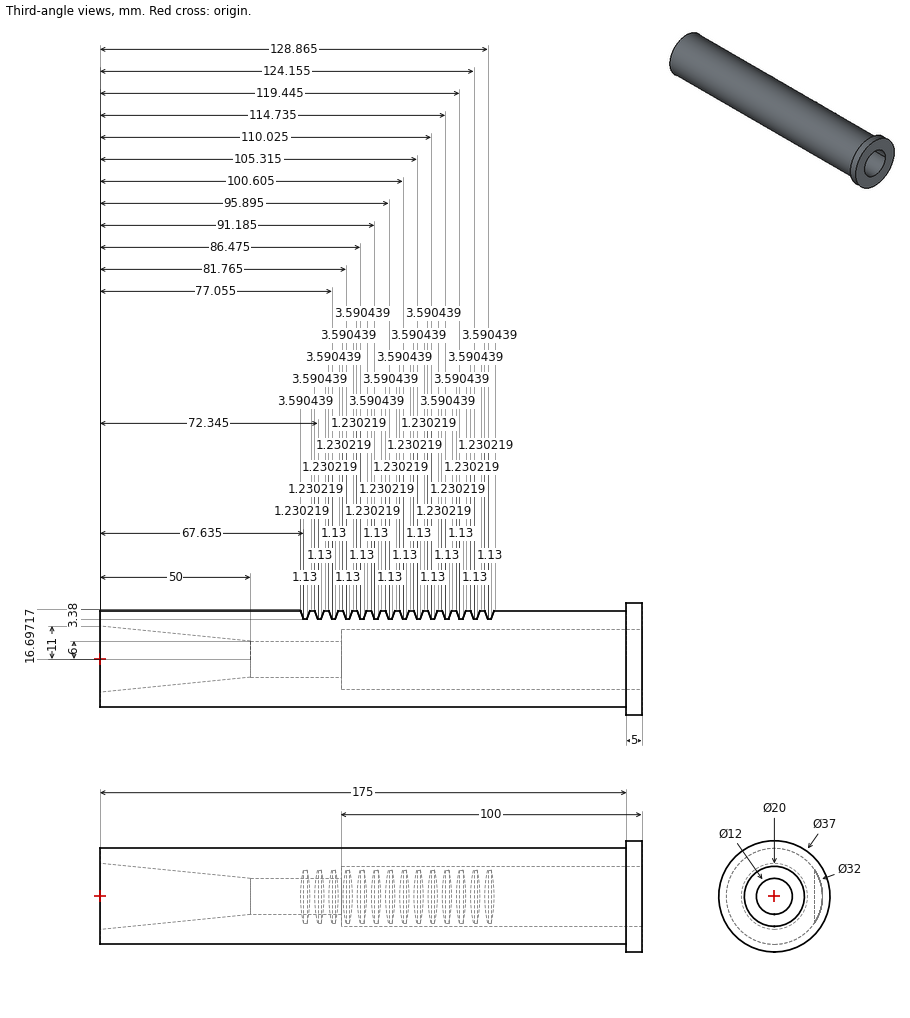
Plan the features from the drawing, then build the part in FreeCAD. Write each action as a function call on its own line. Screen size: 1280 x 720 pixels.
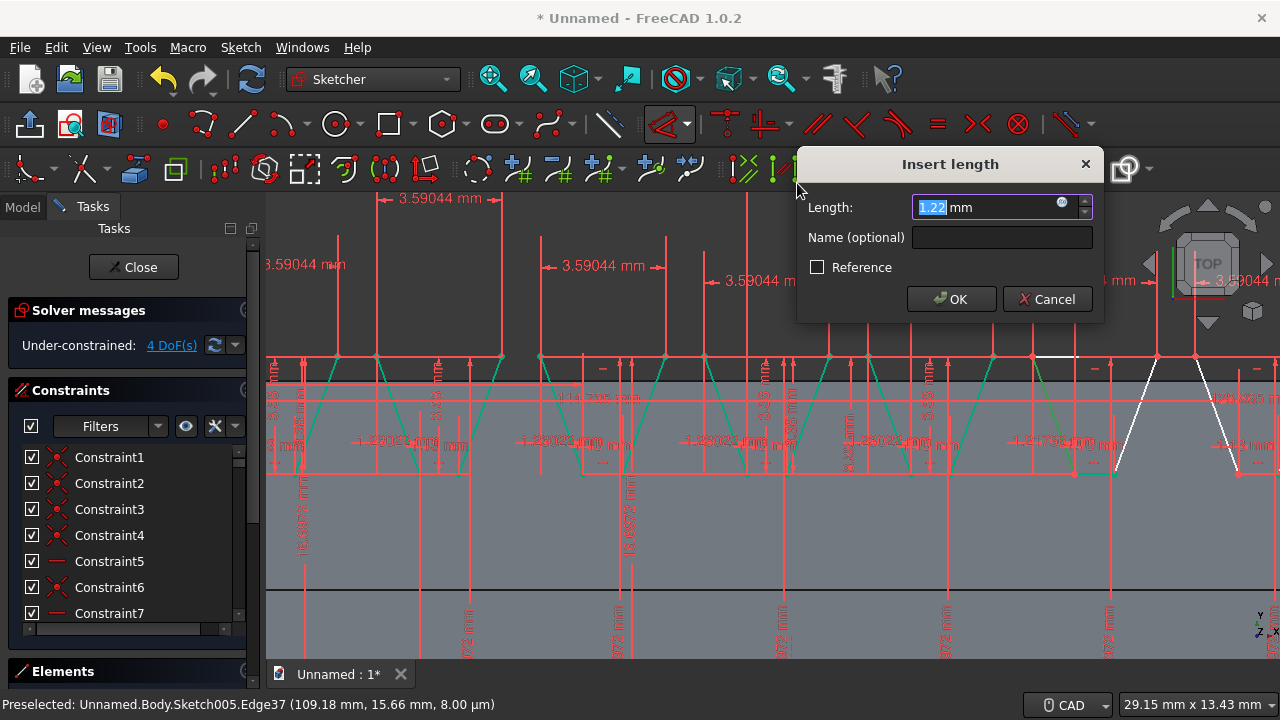
text(1.230219)
key(Return)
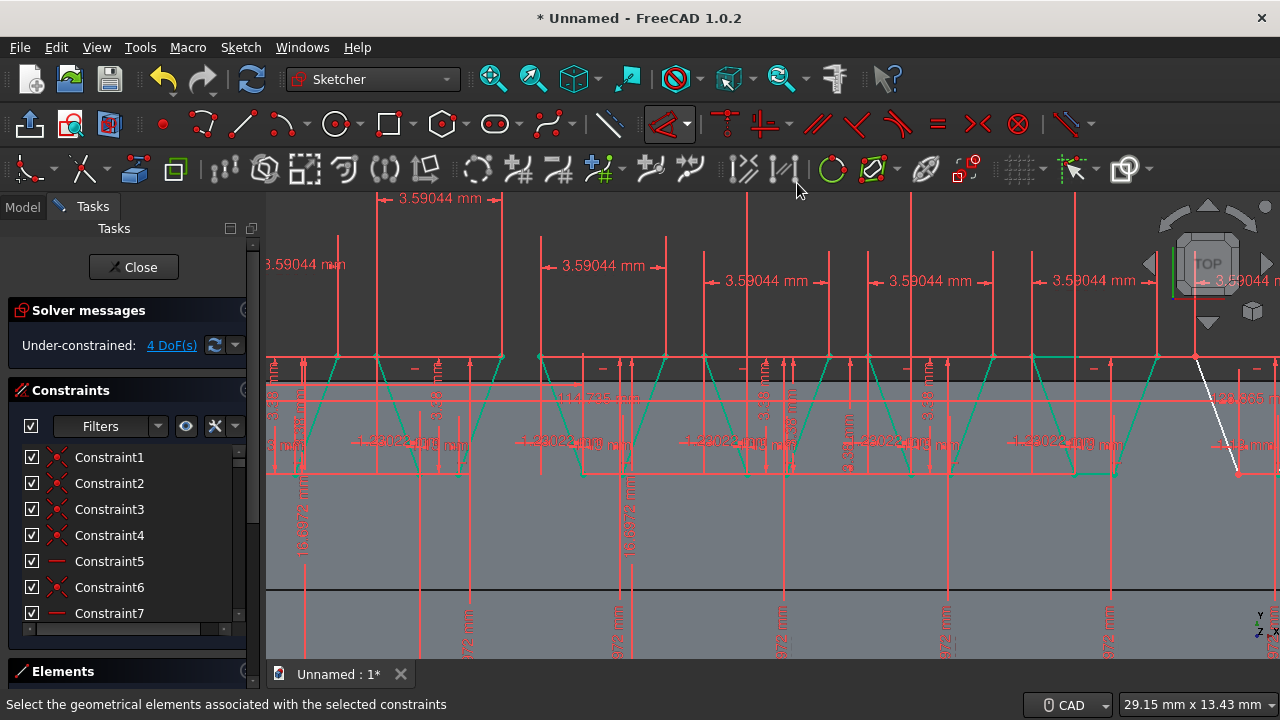
scroll(888, 391, down, 10)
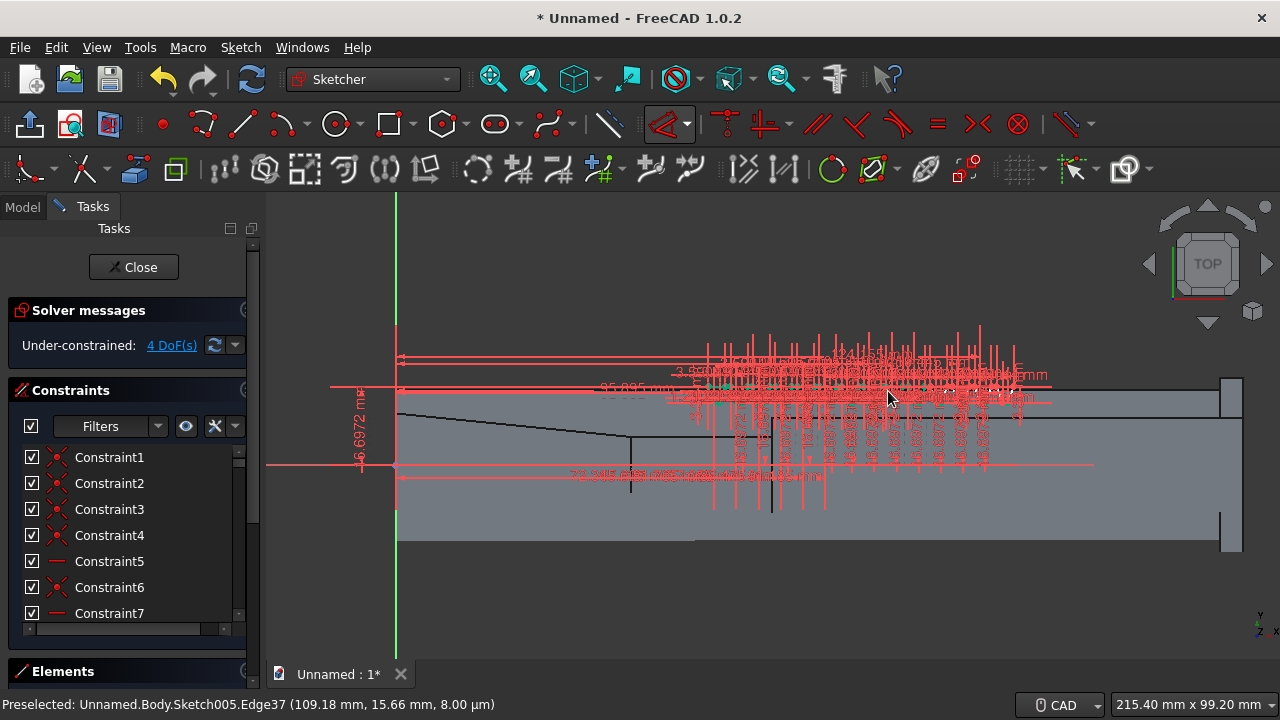
scroll(932, 391, up, 10)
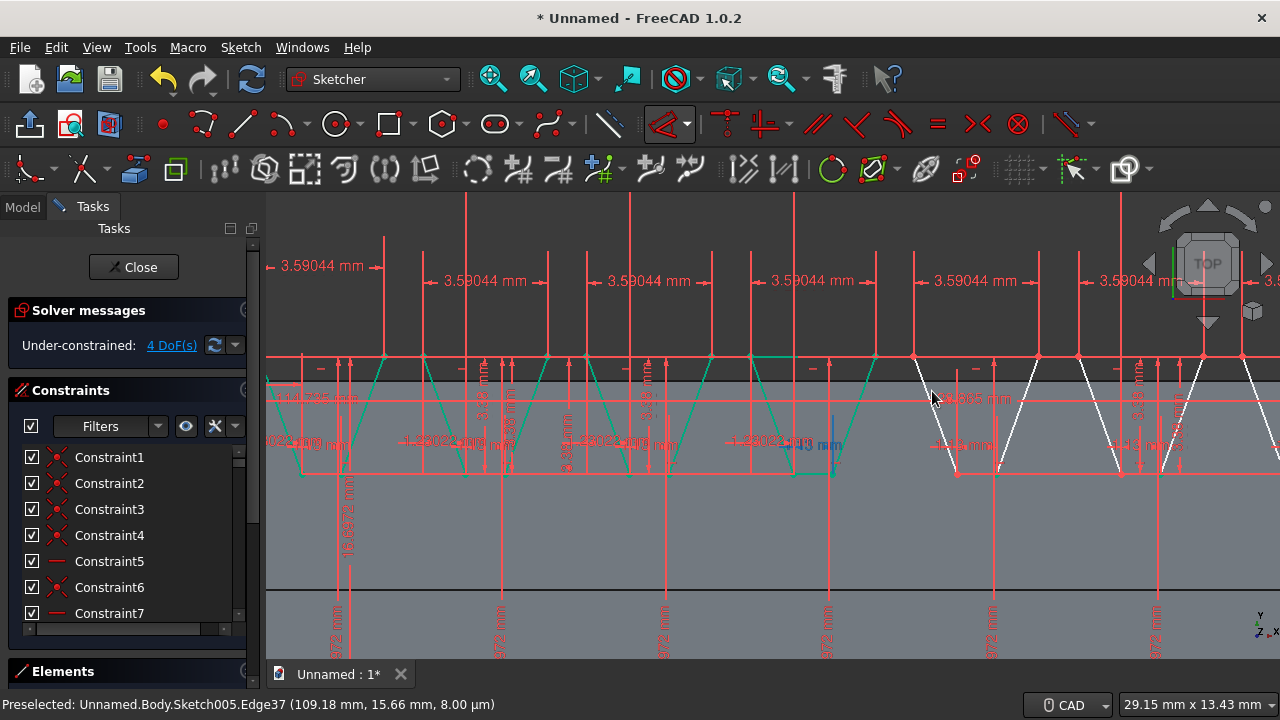
click(927, 392)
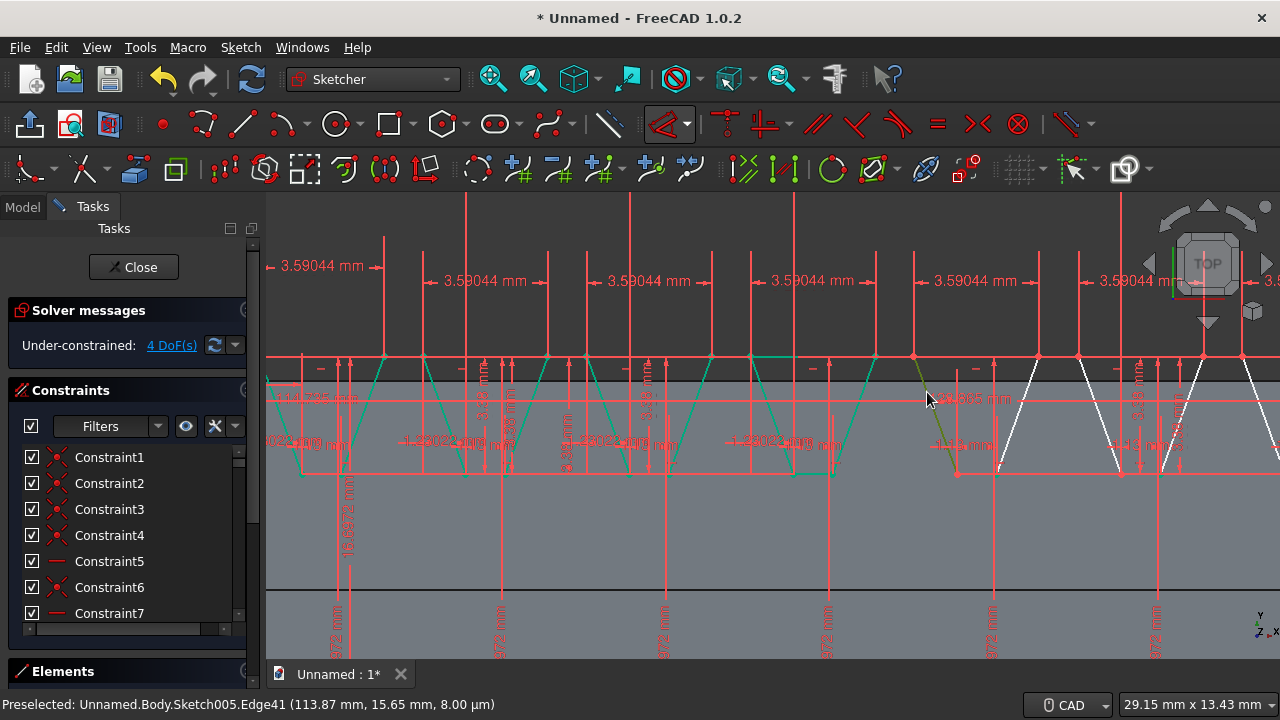
key(l)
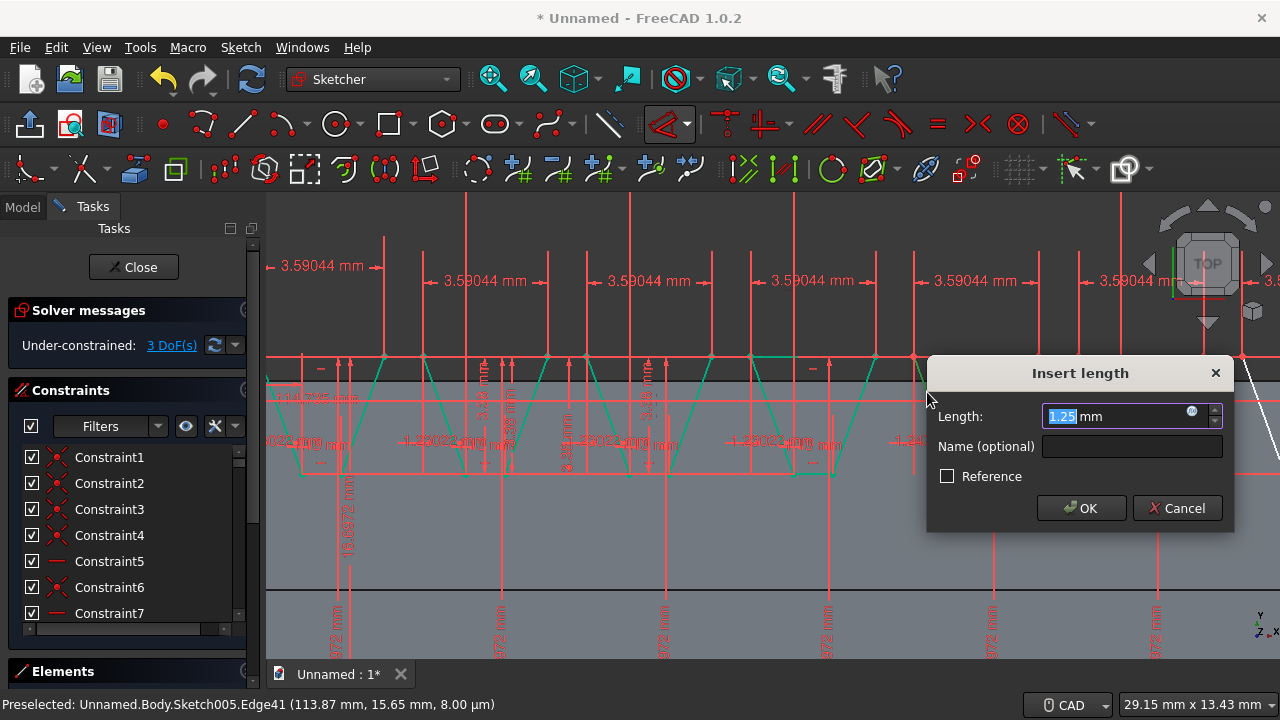
text(1.230219)
key(Return)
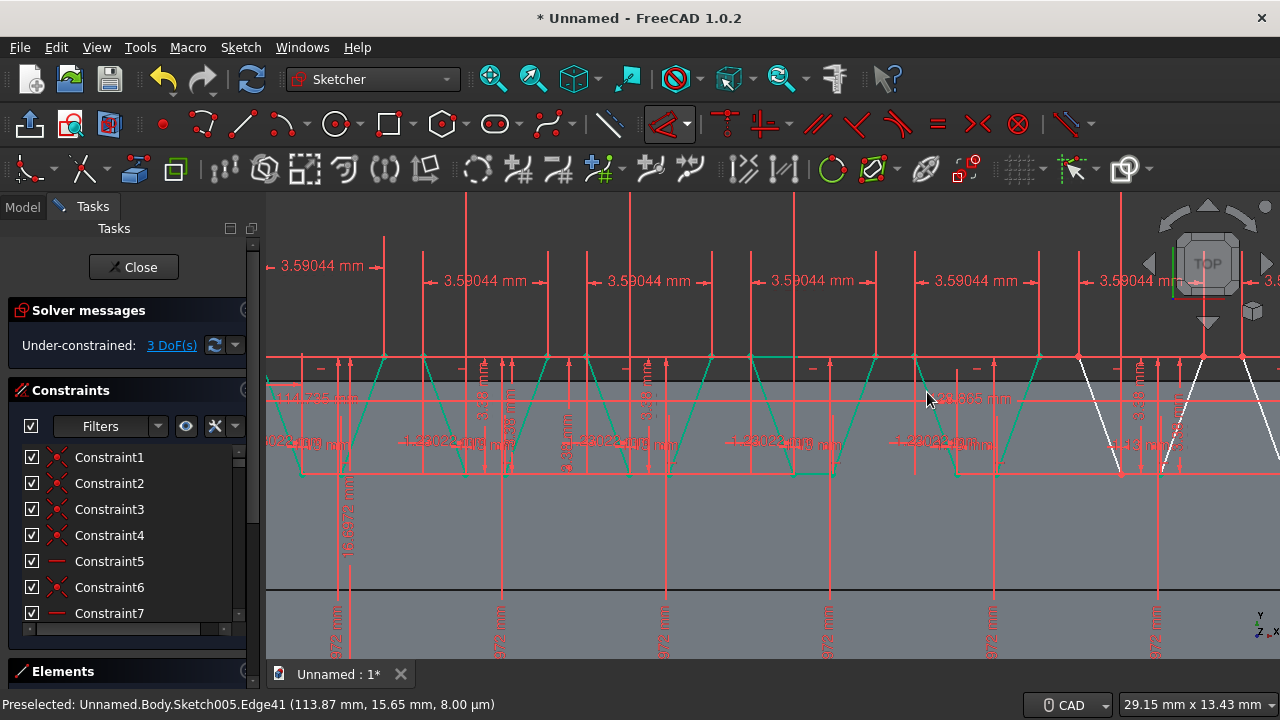
click(1091, 392)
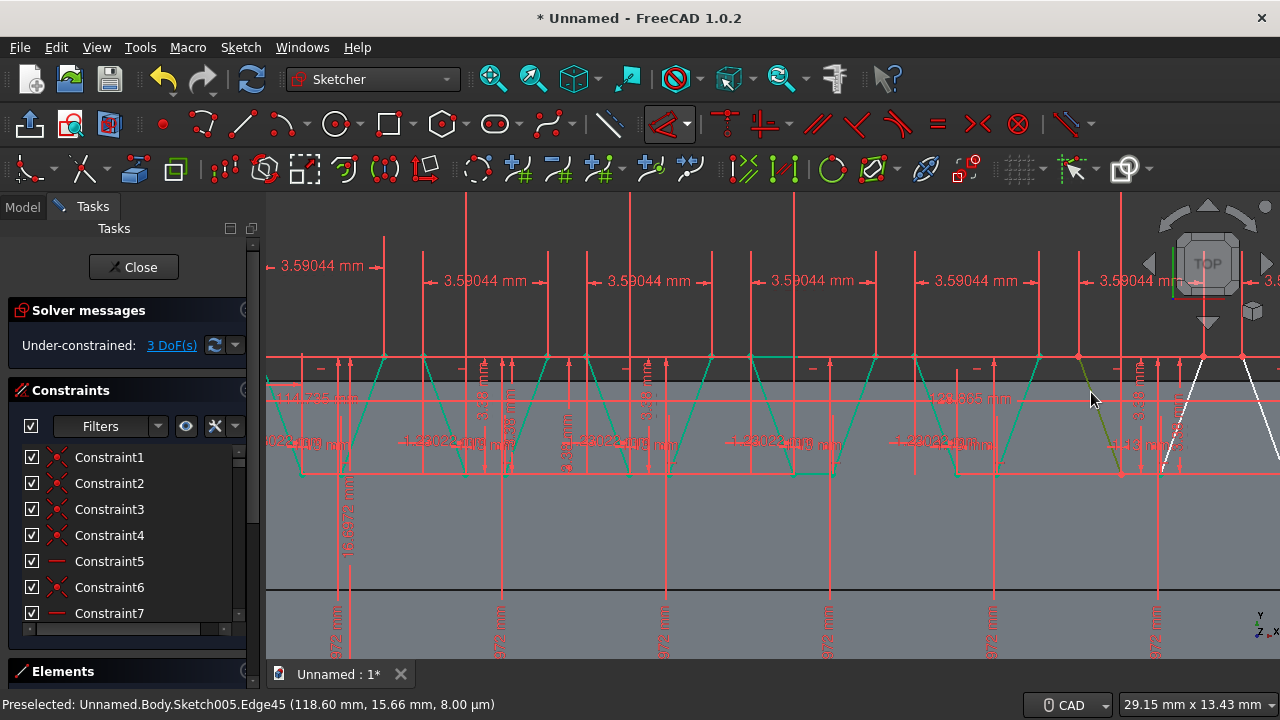
key(l)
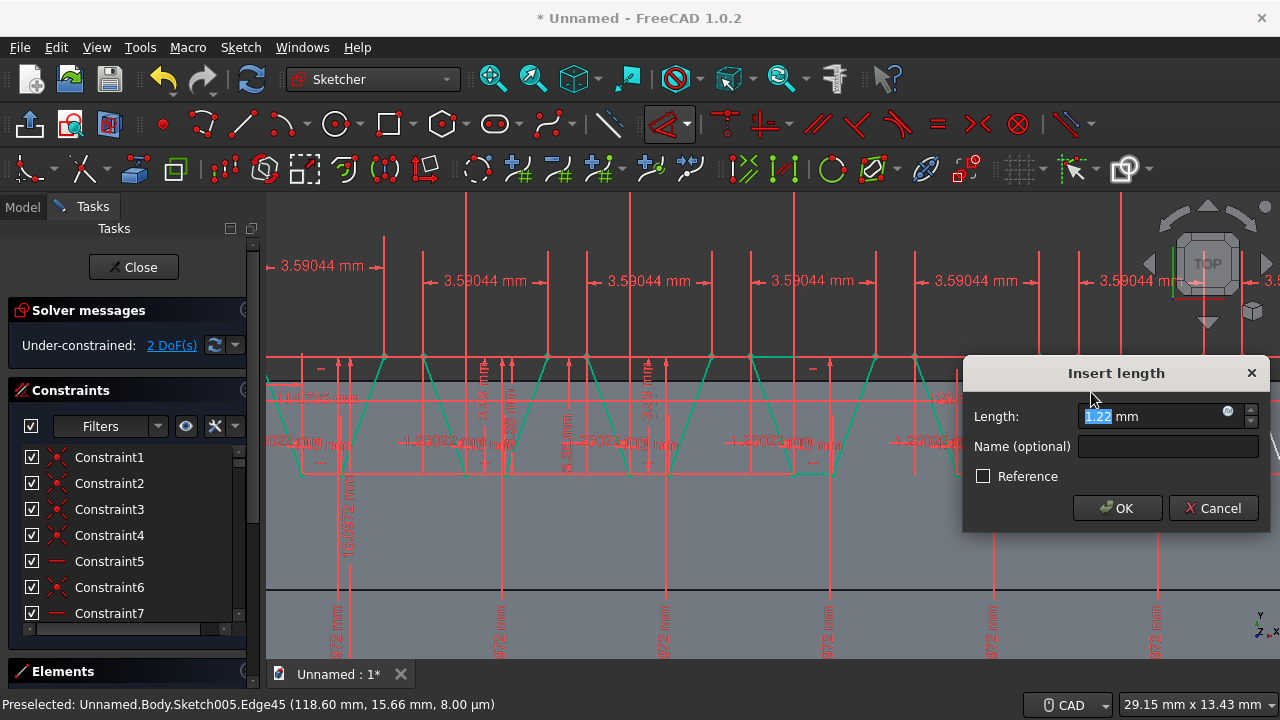
text(1.230219)
key(Return)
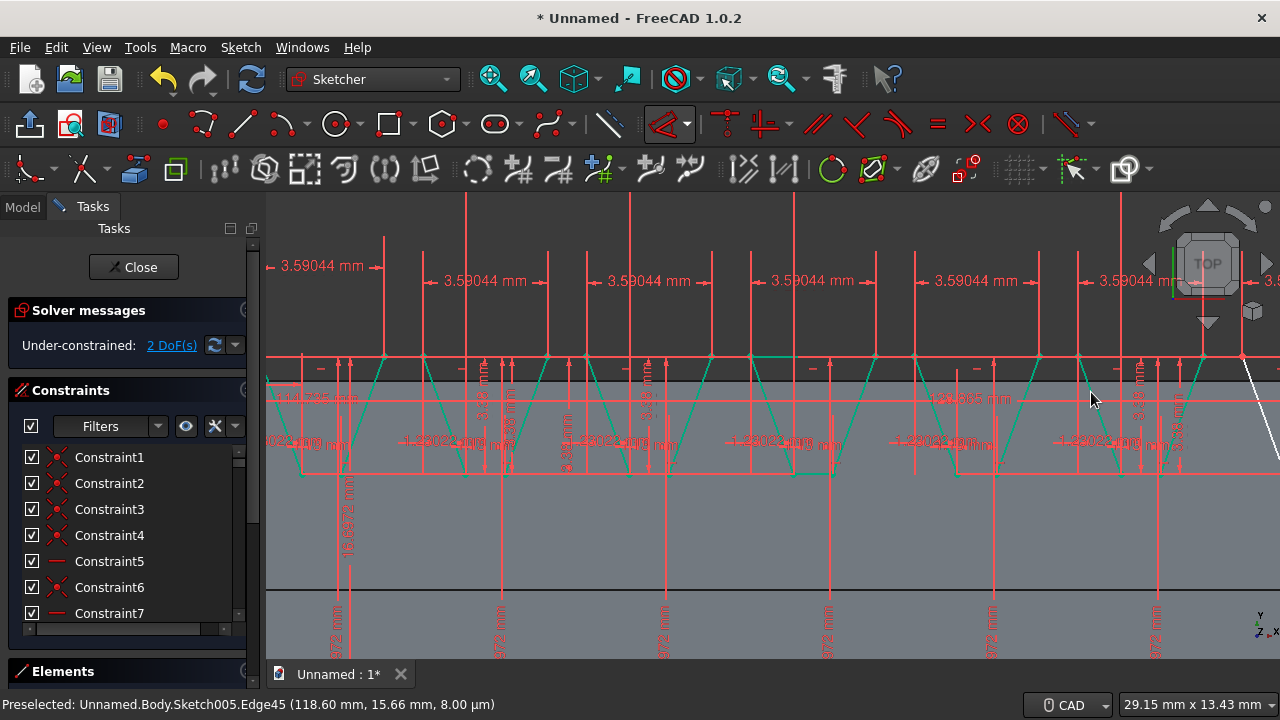
scroll(932, 391, down, 10)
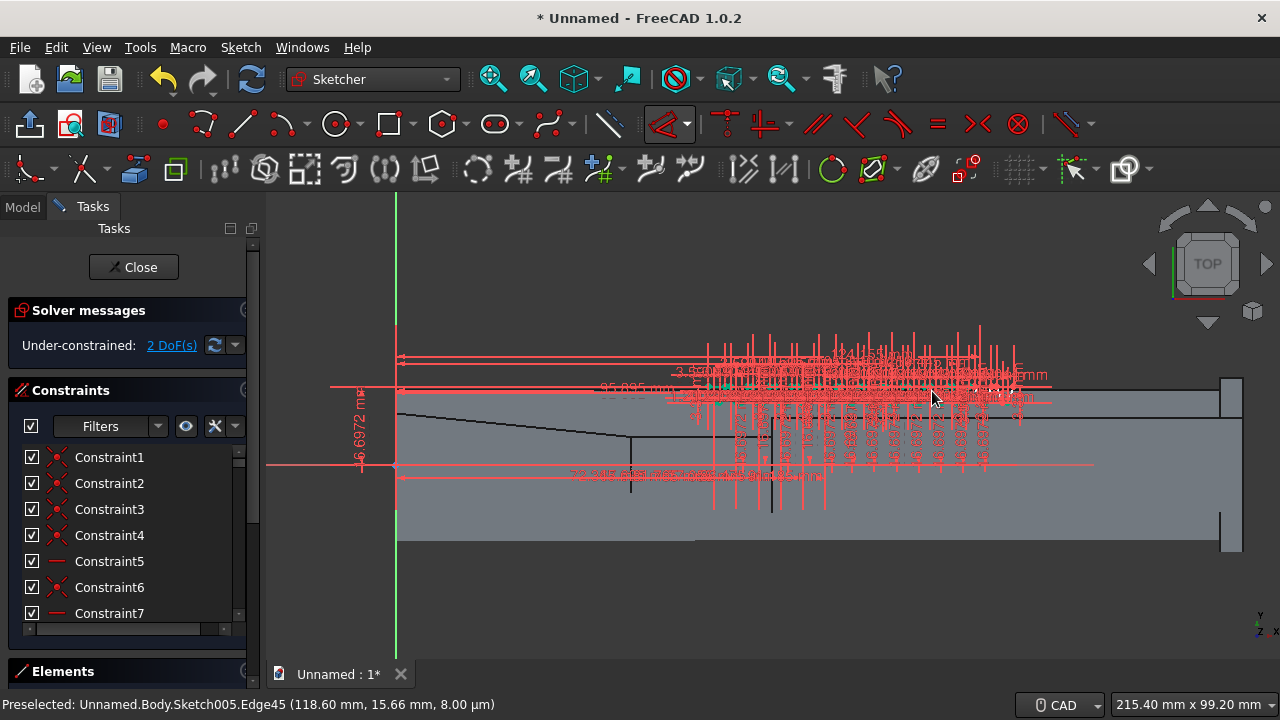
scroll(976, 391, up, 10)